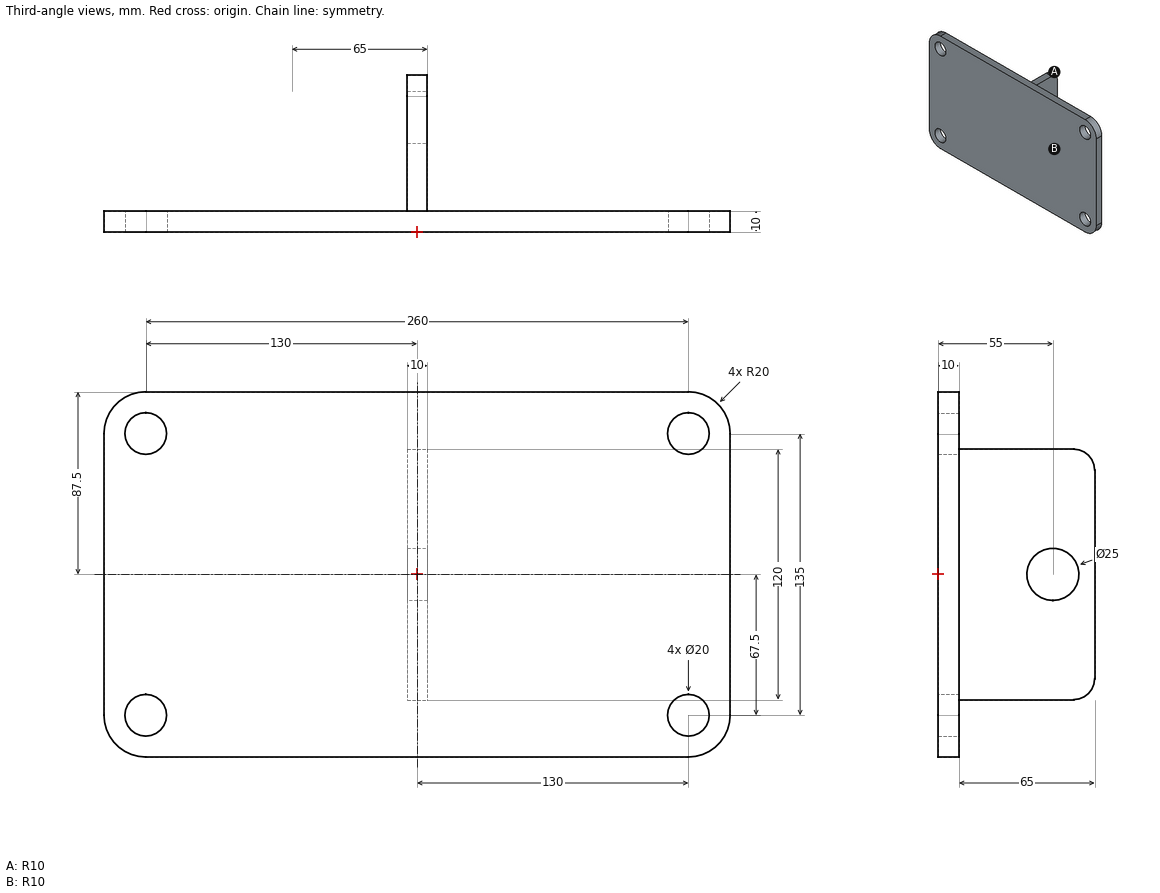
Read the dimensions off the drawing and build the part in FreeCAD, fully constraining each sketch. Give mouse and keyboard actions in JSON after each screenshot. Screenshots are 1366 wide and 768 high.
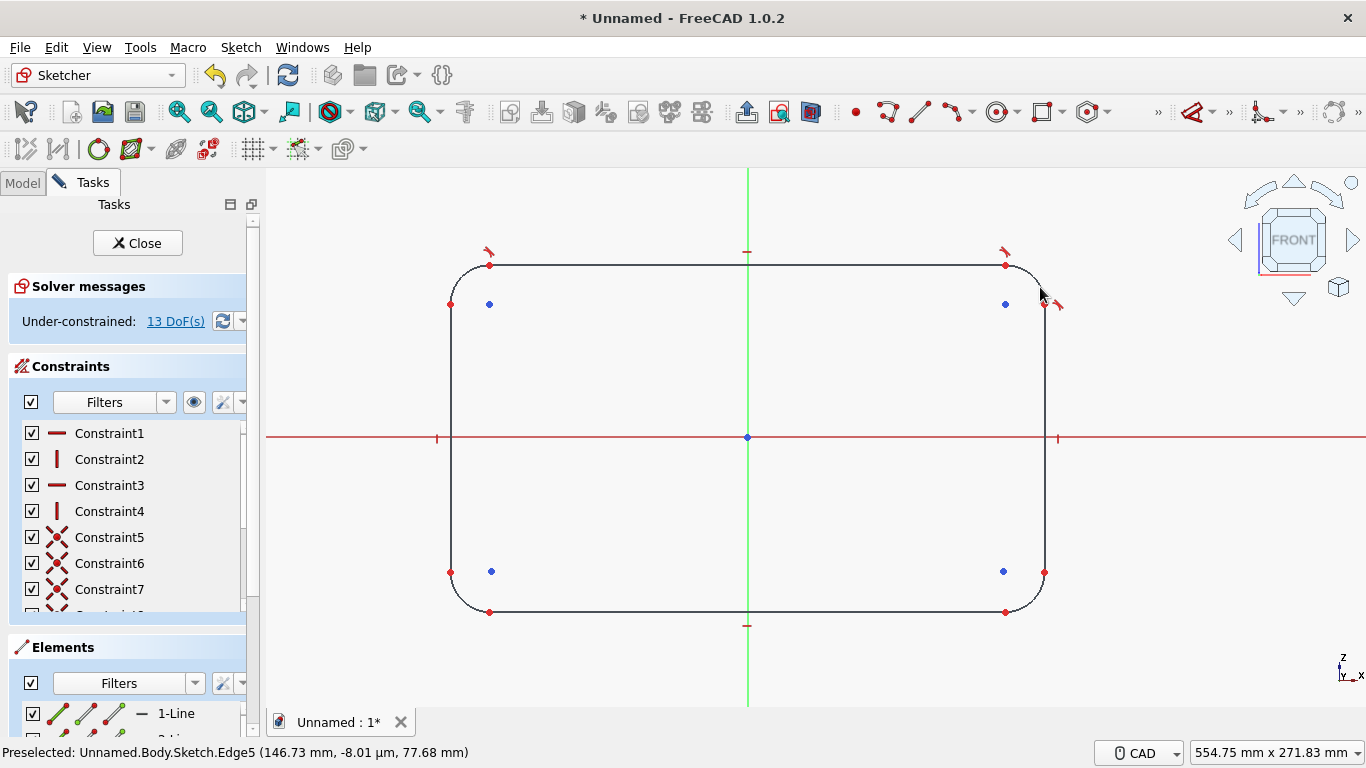
{"action": "left_click", "coordinate": [1045, 385]}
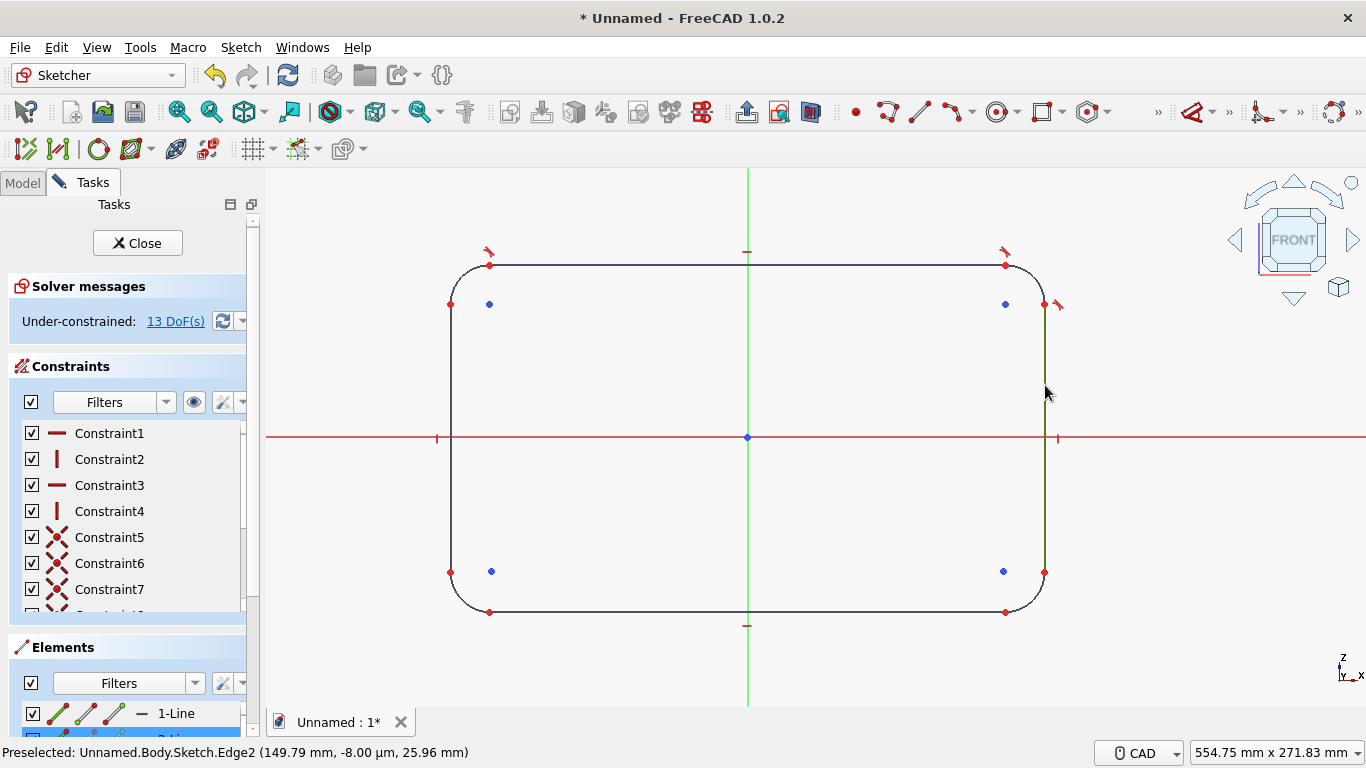
{"action": "left_click", "coordinate": [1023, 607]}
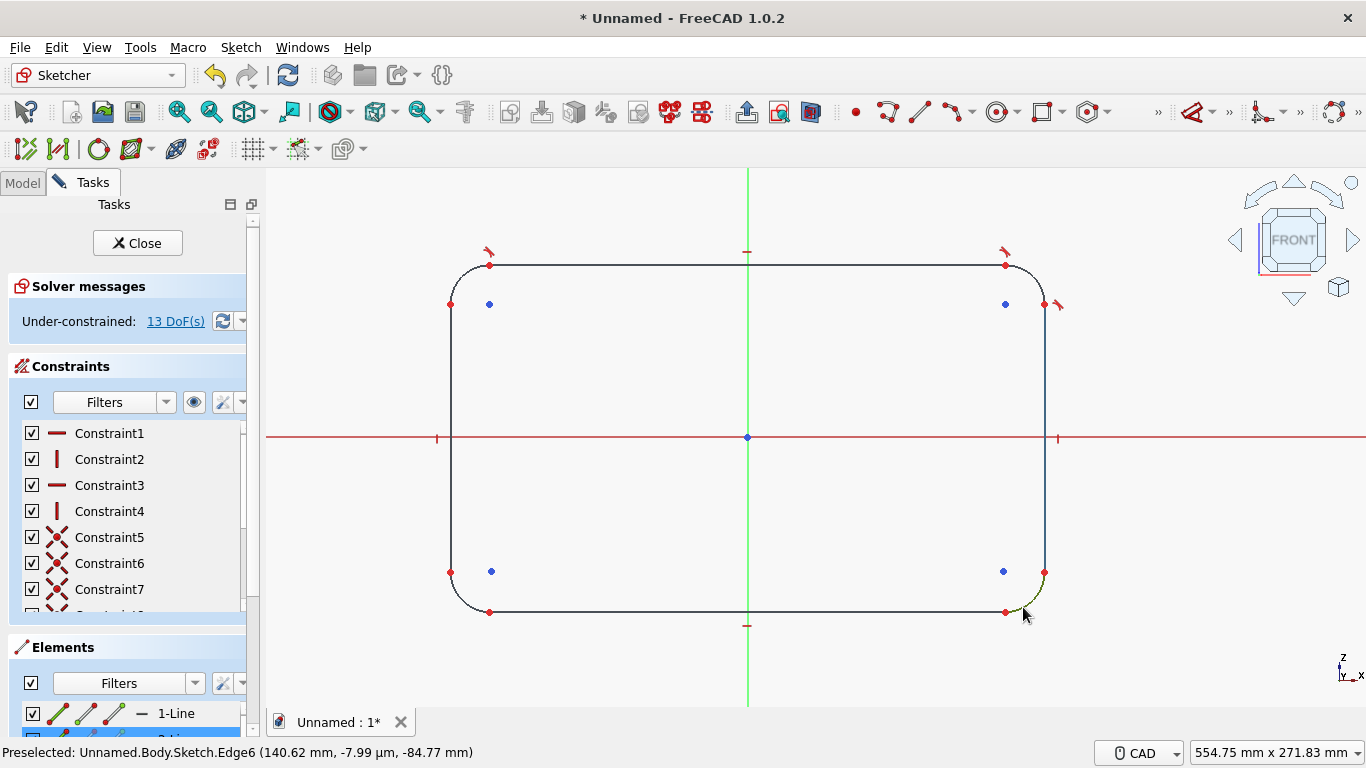
{"action": "key", "text": "t"}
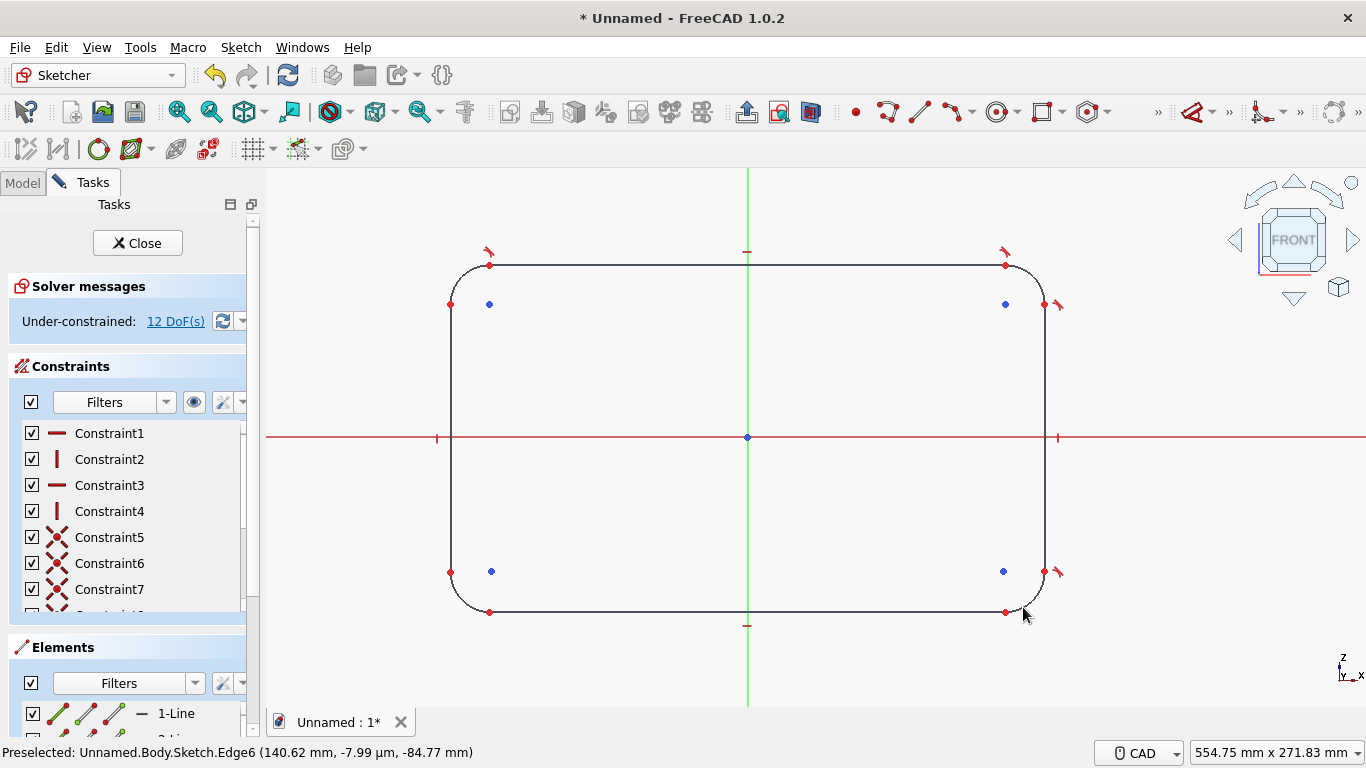
{"action": "left_click", "coordinate": [851, 612]}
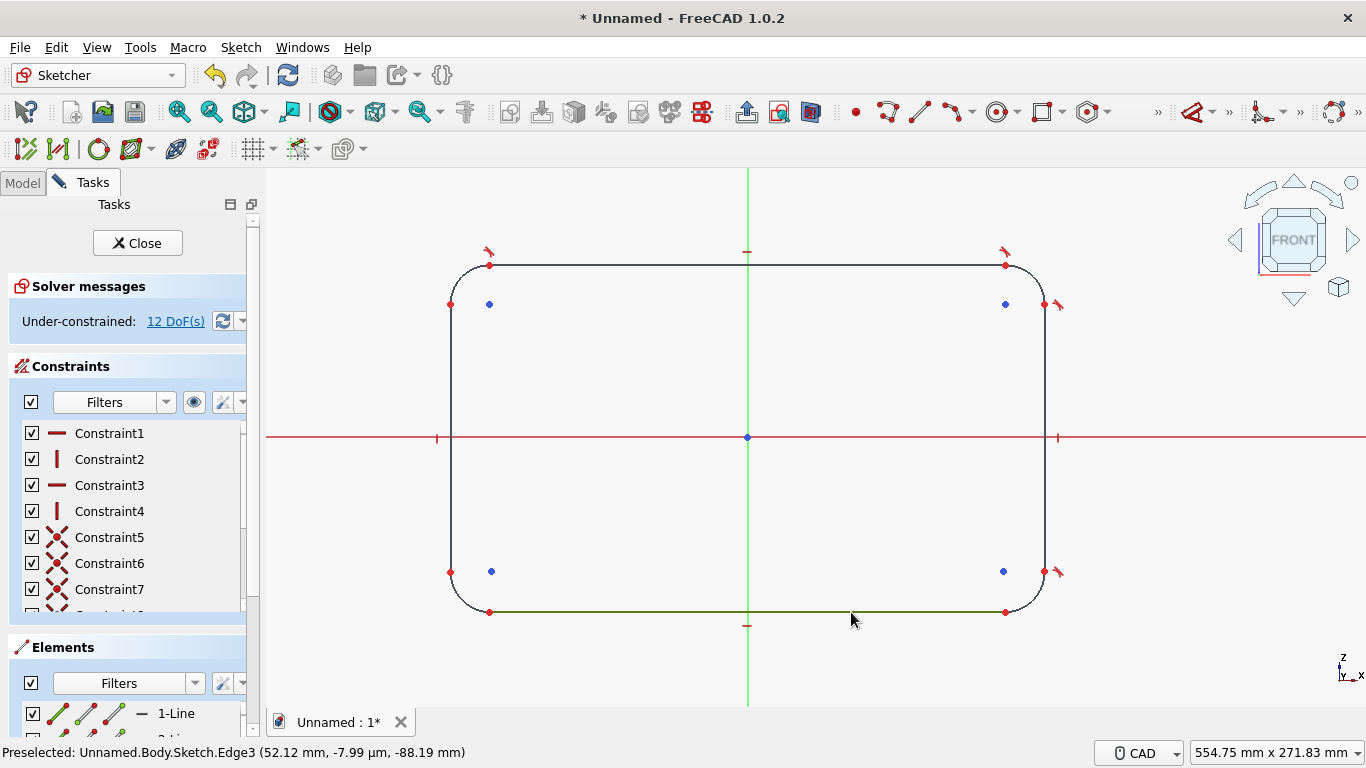
{"action": "left_click", "coordinate": [1024, 607]}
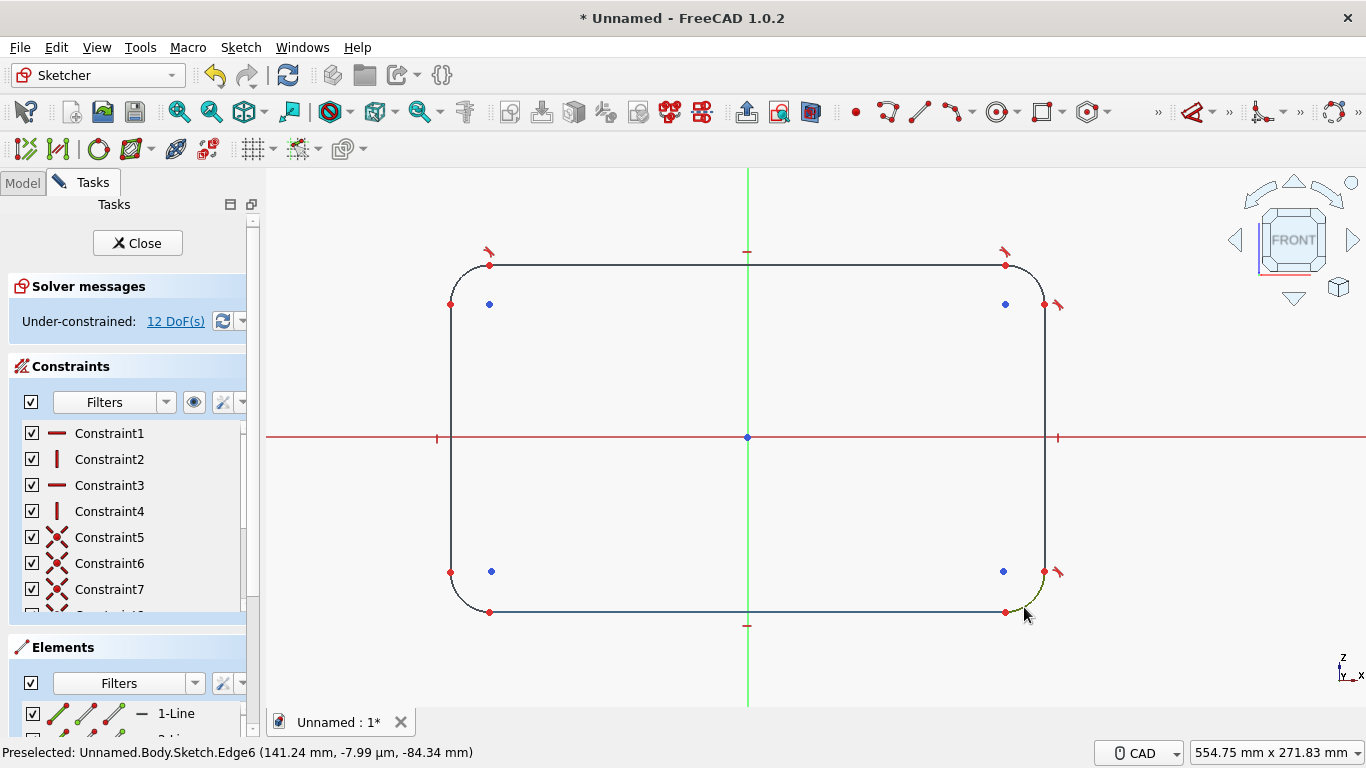
{"action": "key", "text": "t"}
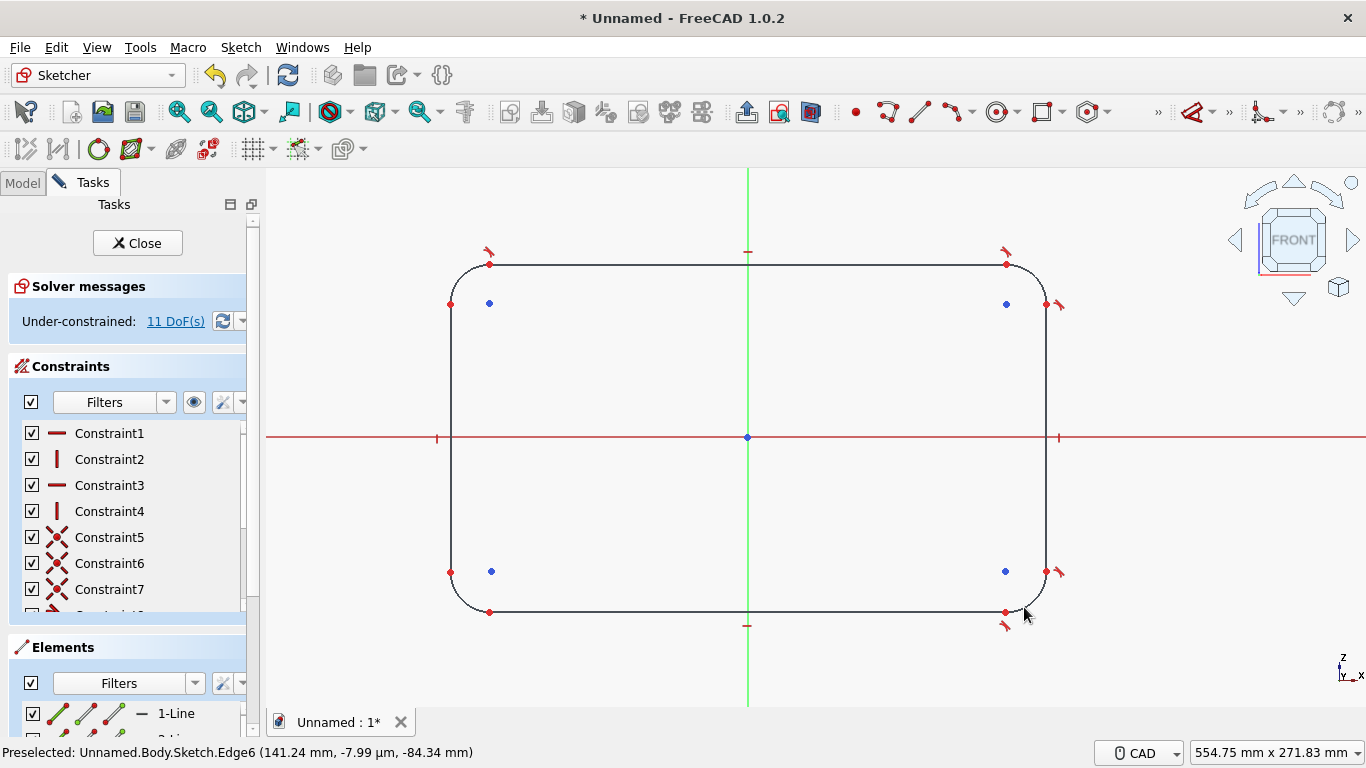
{"action": "left_click", "coordinate": [851, 612]}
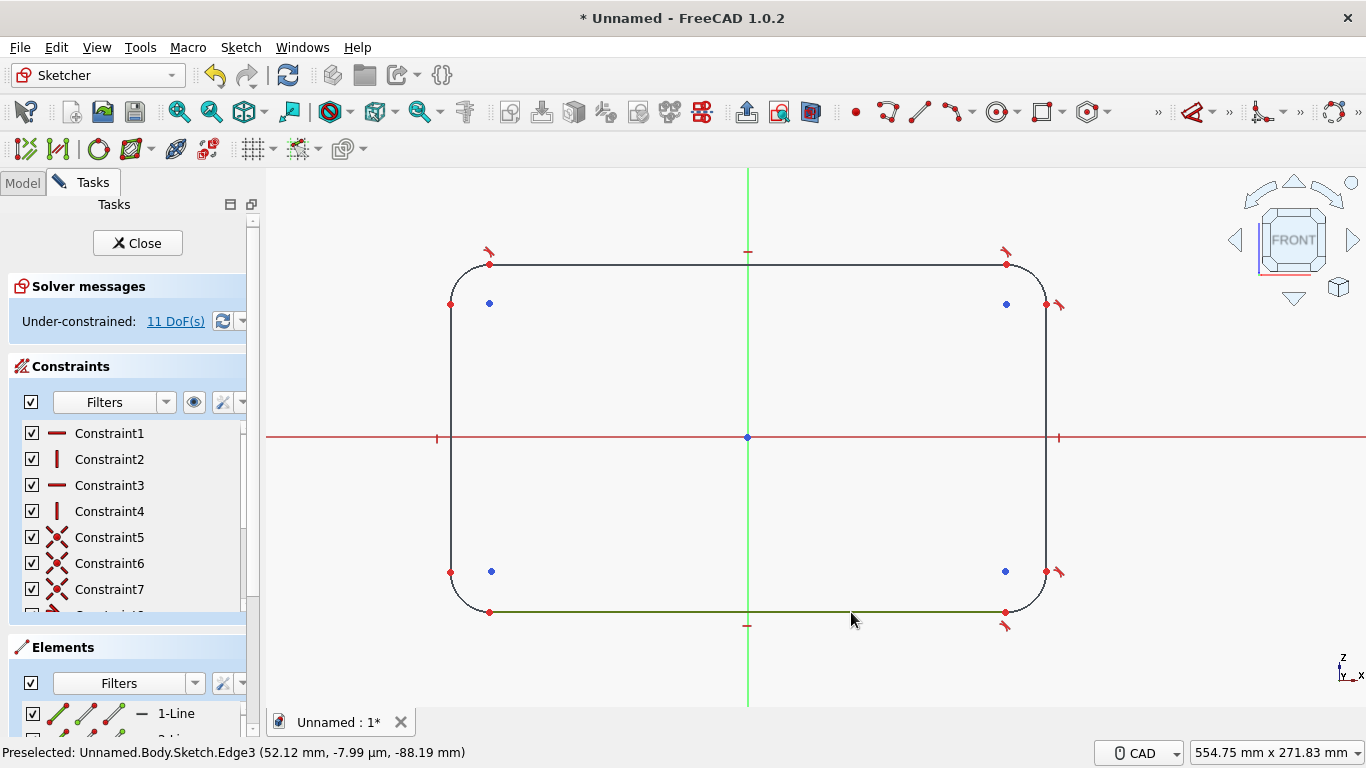
{"action": "left_click", "coordinate": [455, 590]}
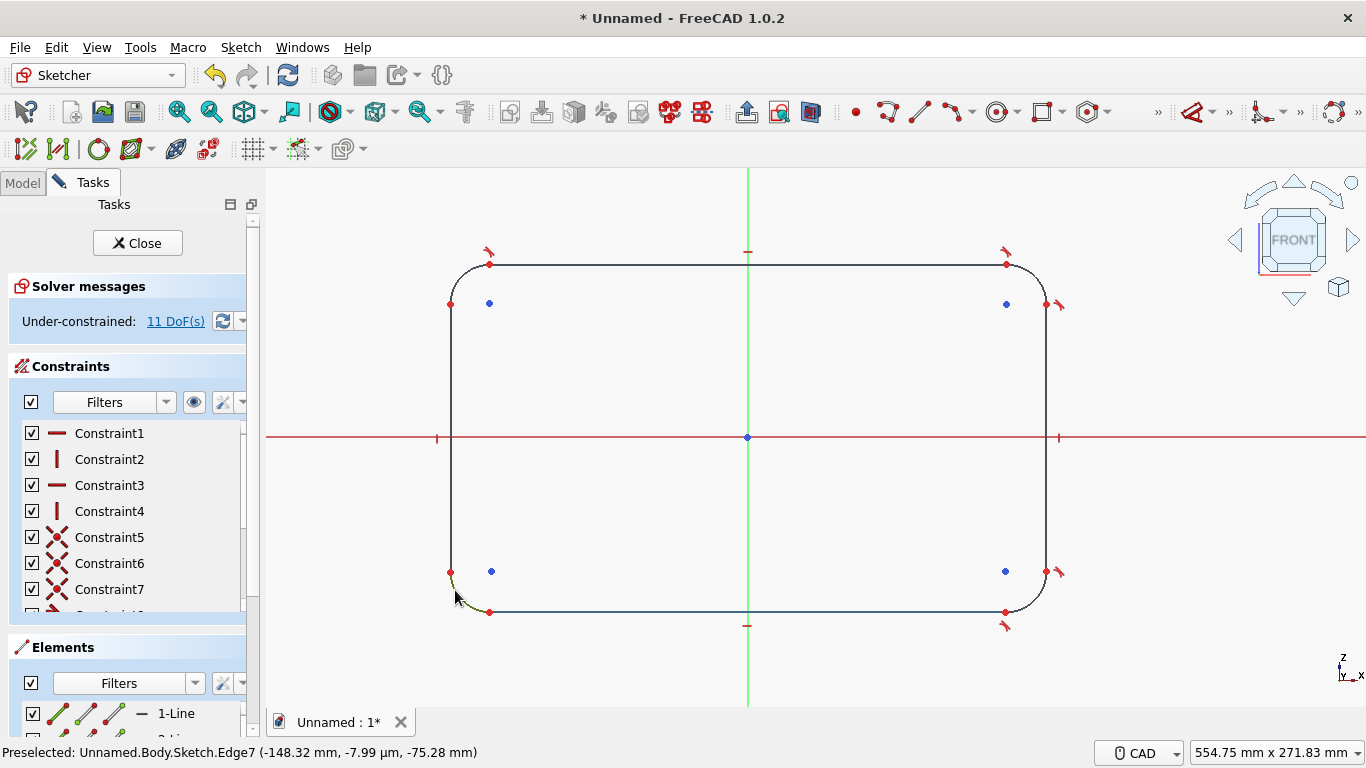
{"action": "key", "text": "t"}